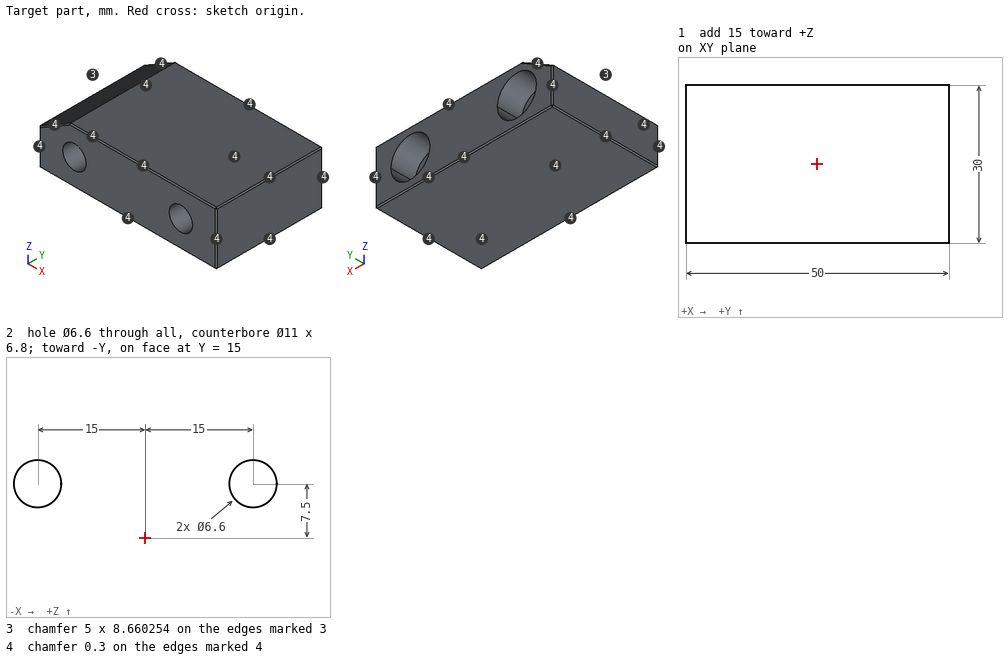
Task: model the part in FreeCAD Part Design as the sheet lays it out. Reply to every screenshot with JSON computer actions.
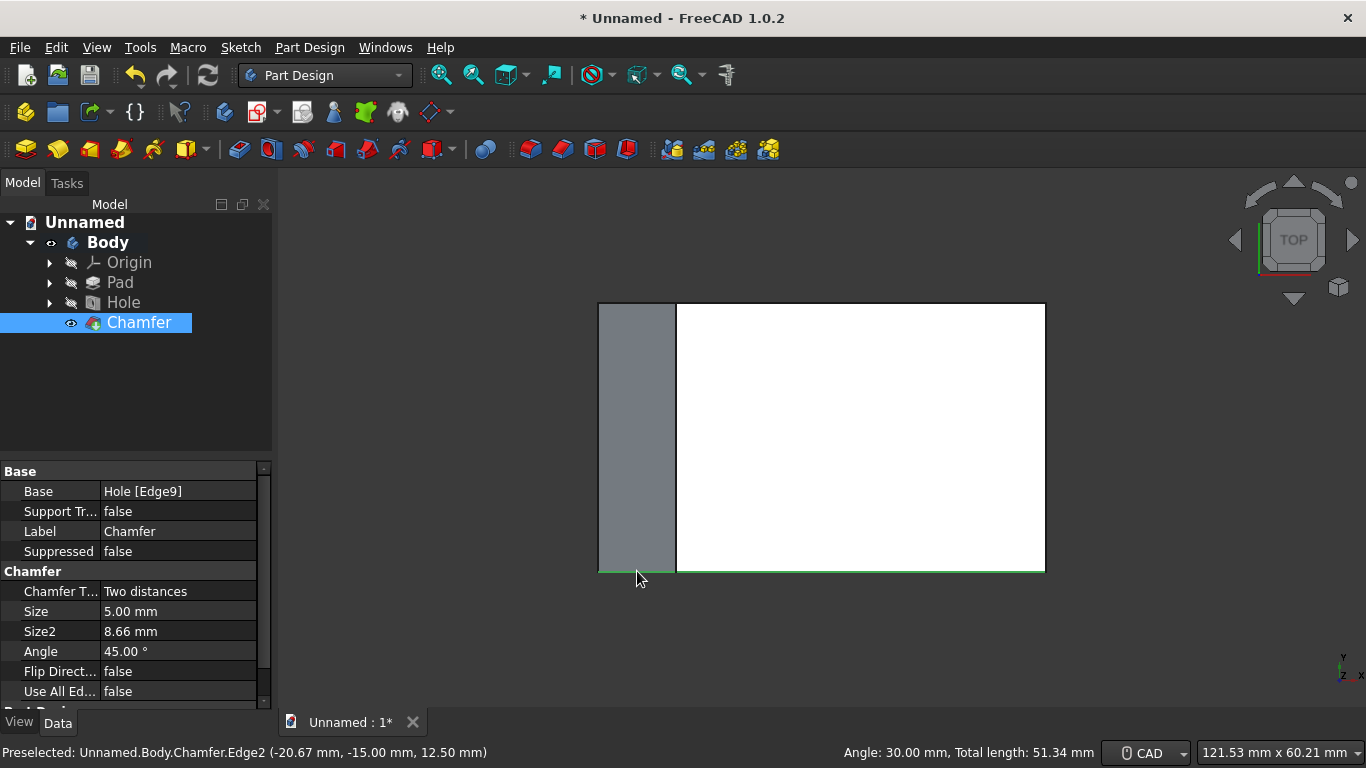
{"action": "left_click", "coordinate": [637, 302], "text": "ctrl"}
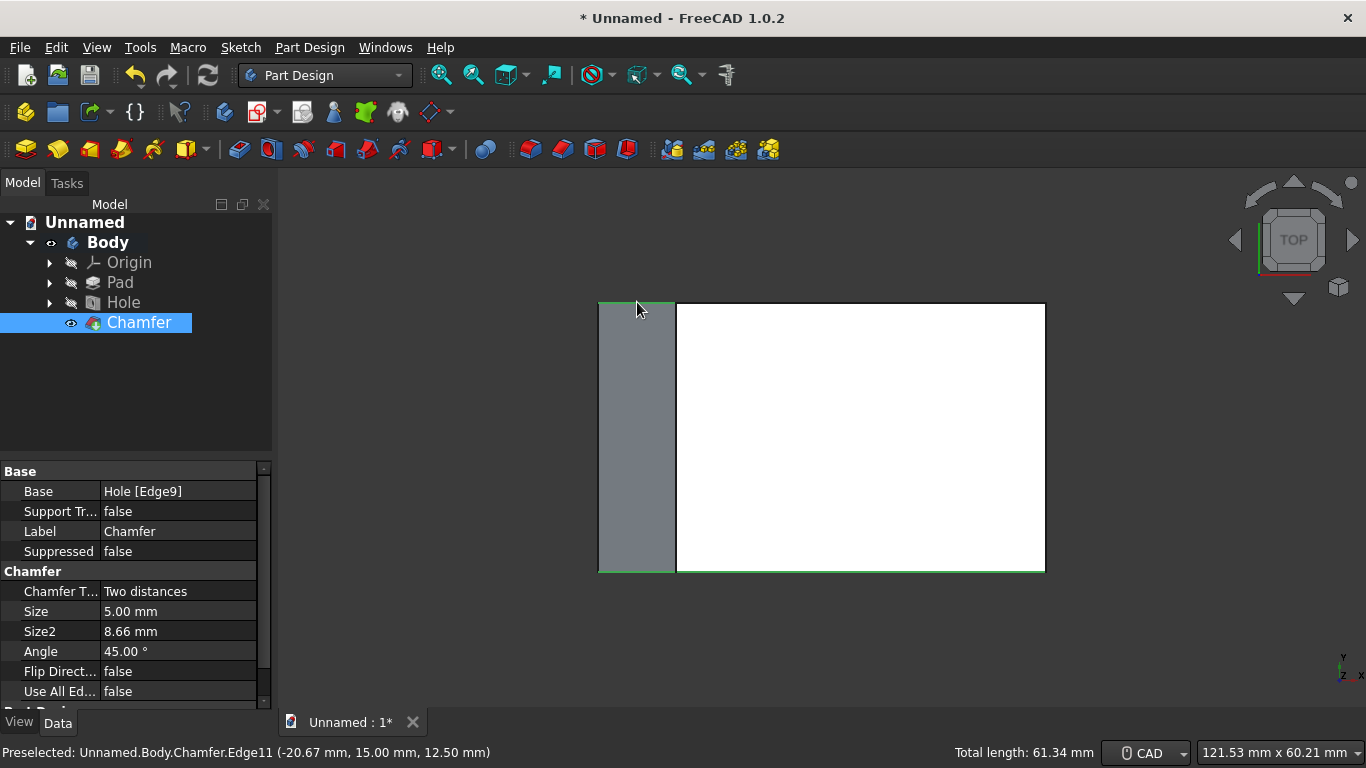
{"action": "left_click", "coordinate": [861, 302], "text": "ctrl"}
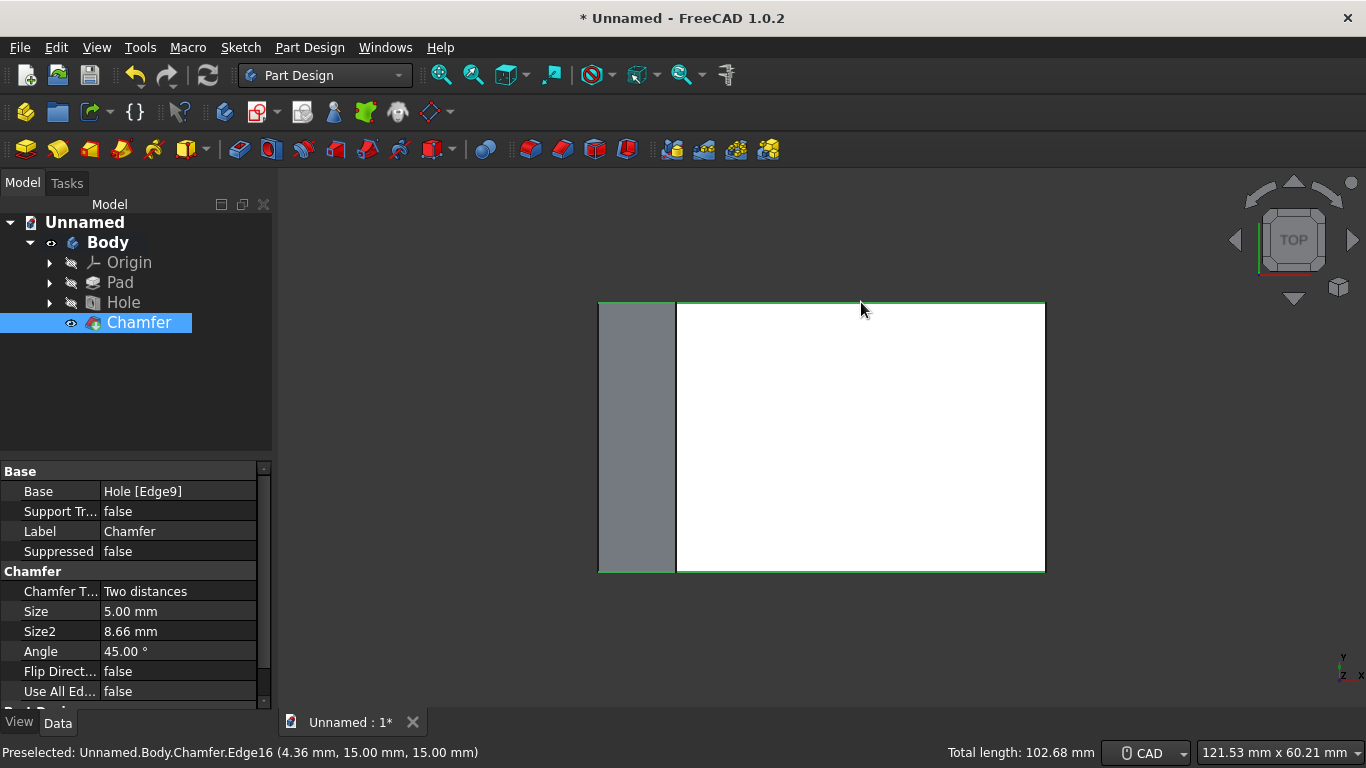
{"action": "key", "text": "0"}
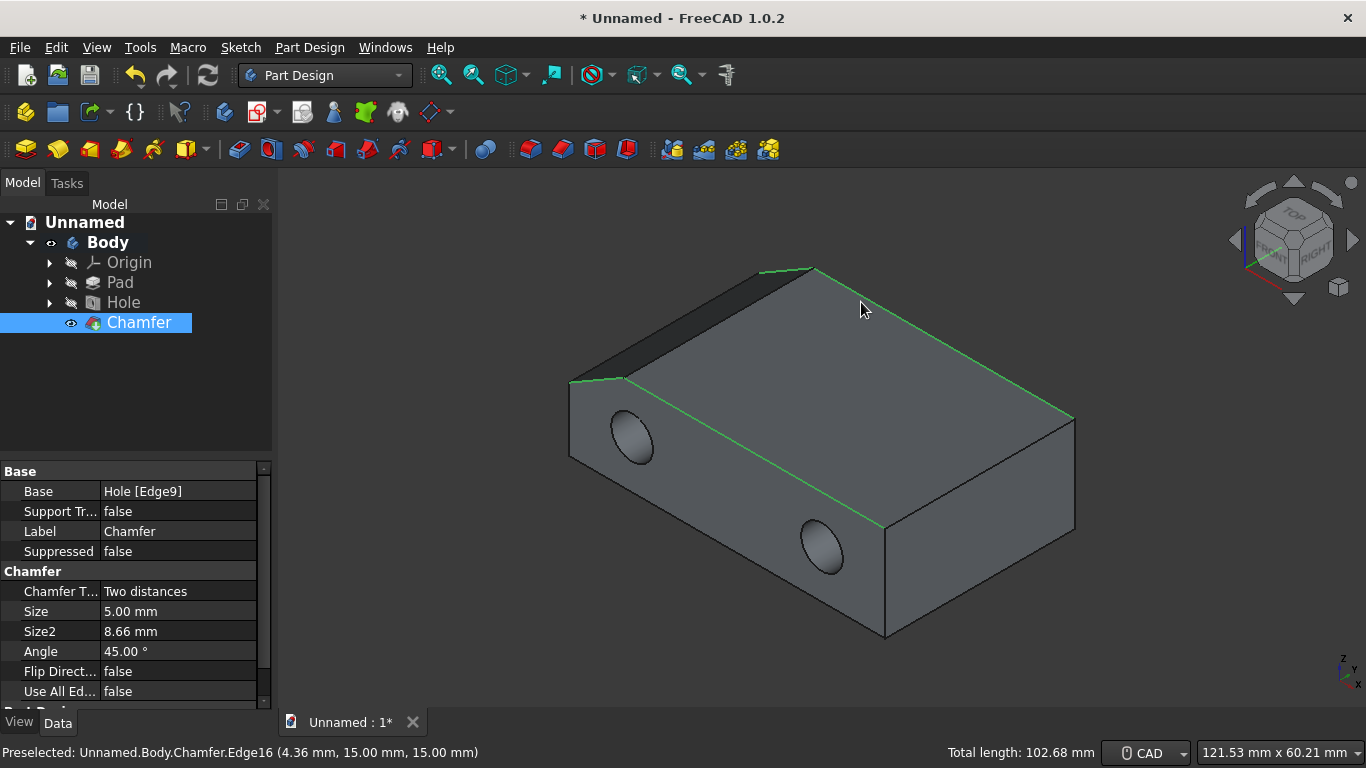
{"action": "left_click", "coordinate": [1007, 512], "text": "ctrl"}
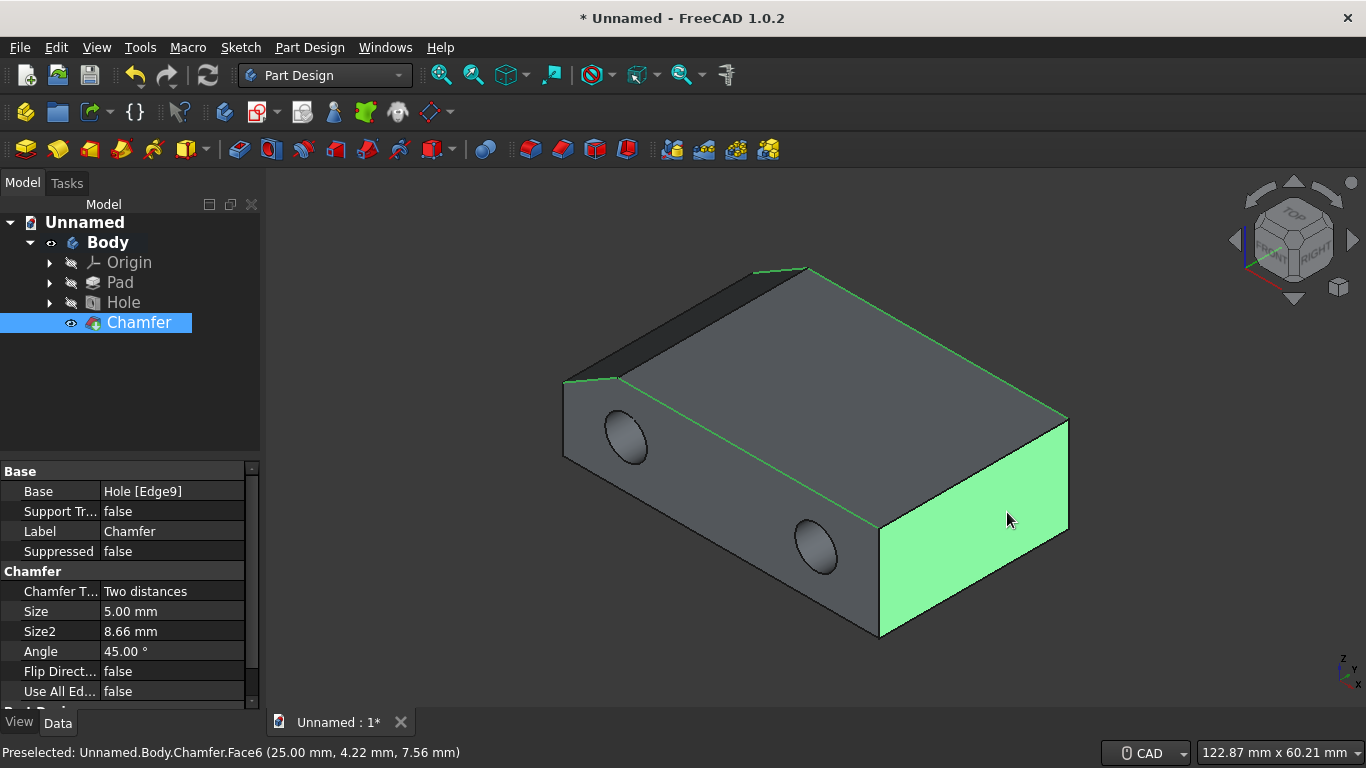
{"action": "key", "text": "2"}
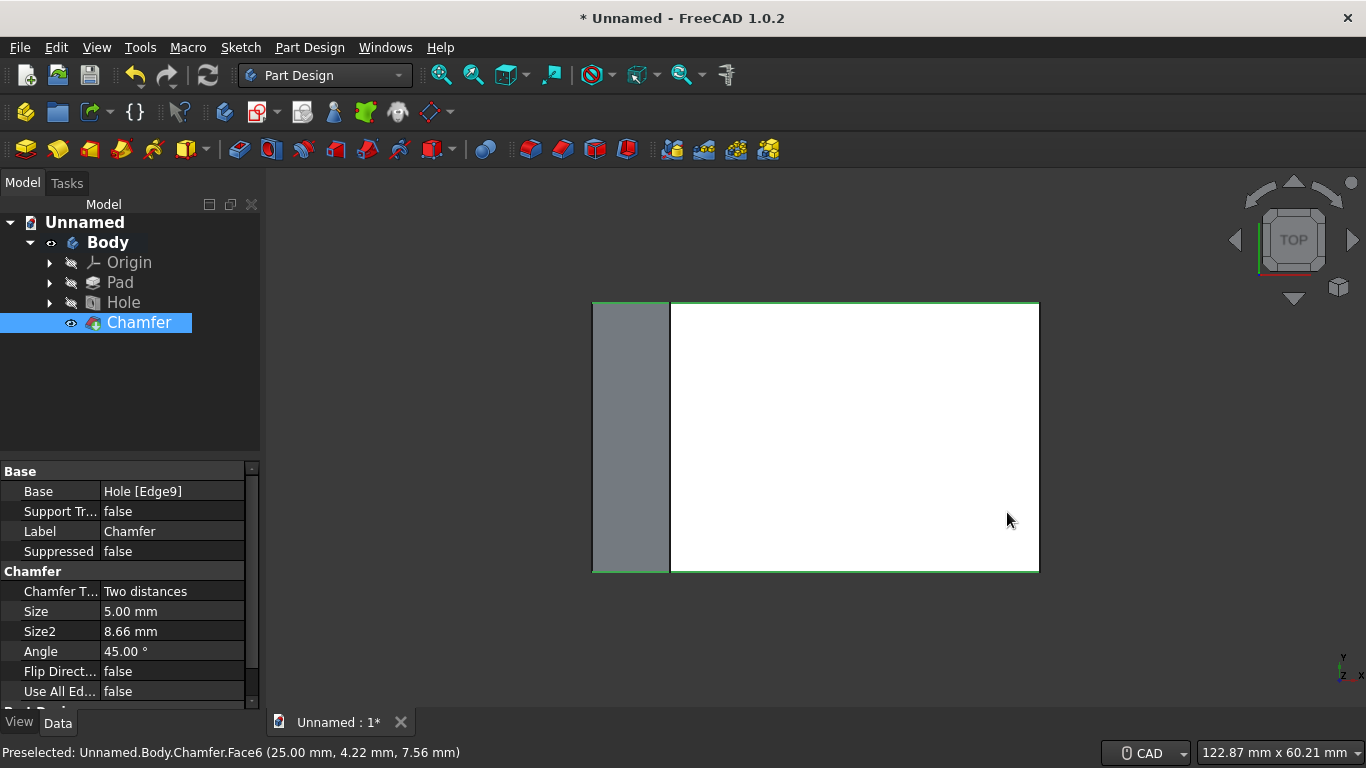
{"action": "key", "text": "1"}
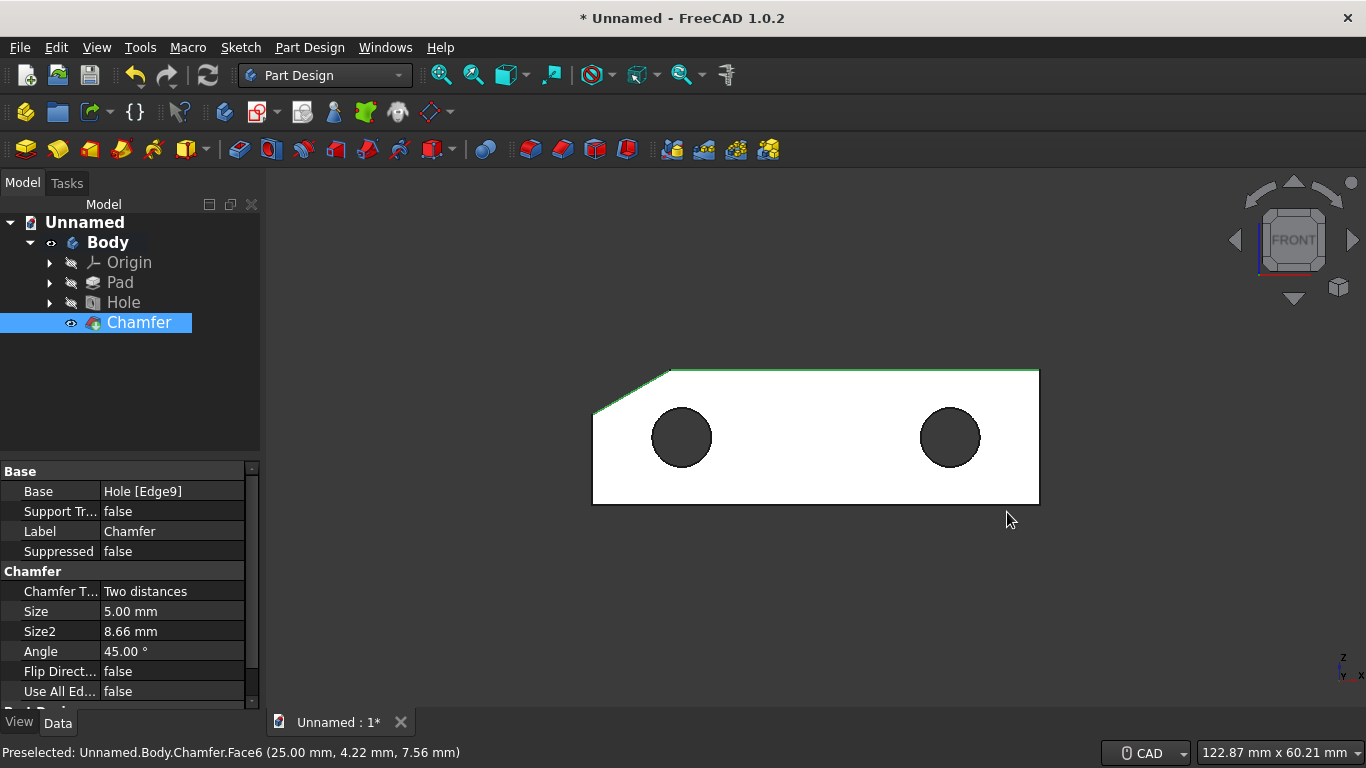
{"action": "left_click", "coordinate": [442, 76]}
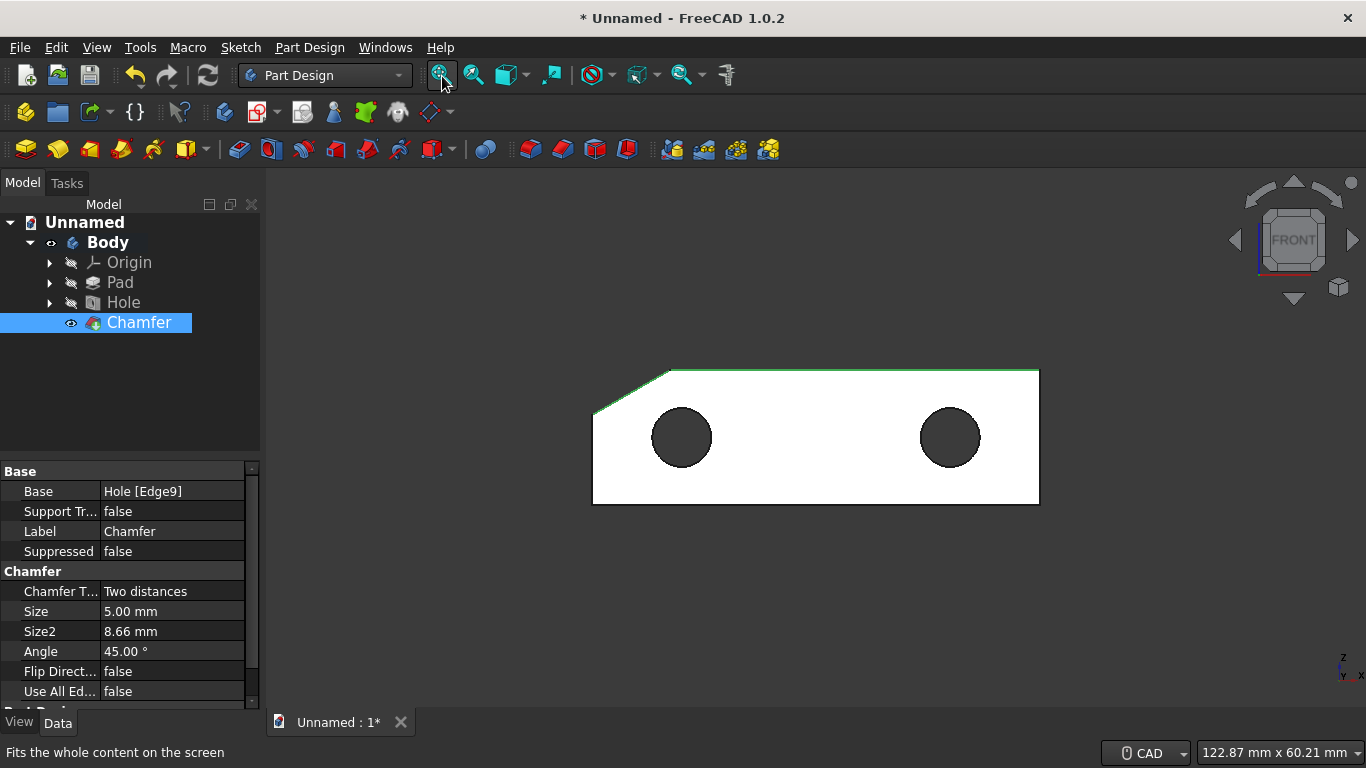
{"action": "left_click", "coordinate": [592, 459], "text": "ctrl"}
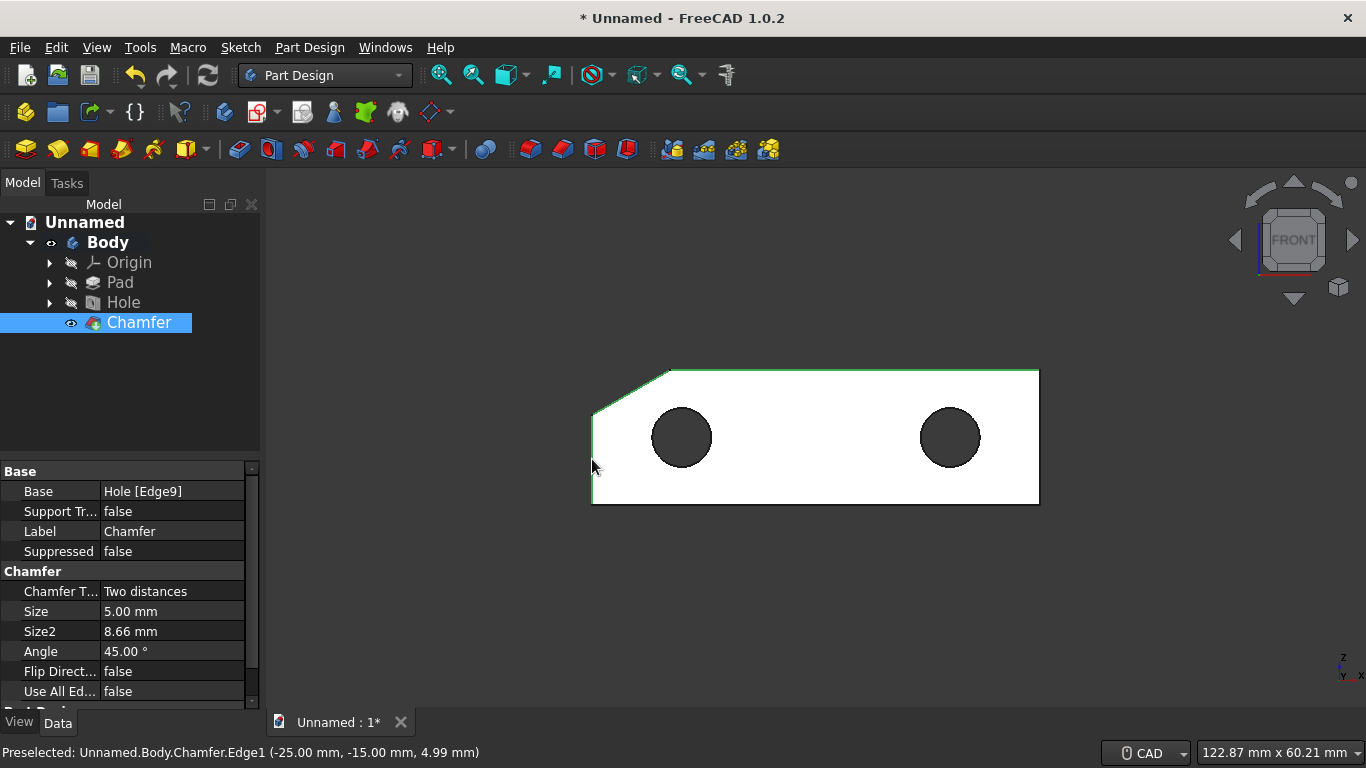
{"action": "key", "text": "3"}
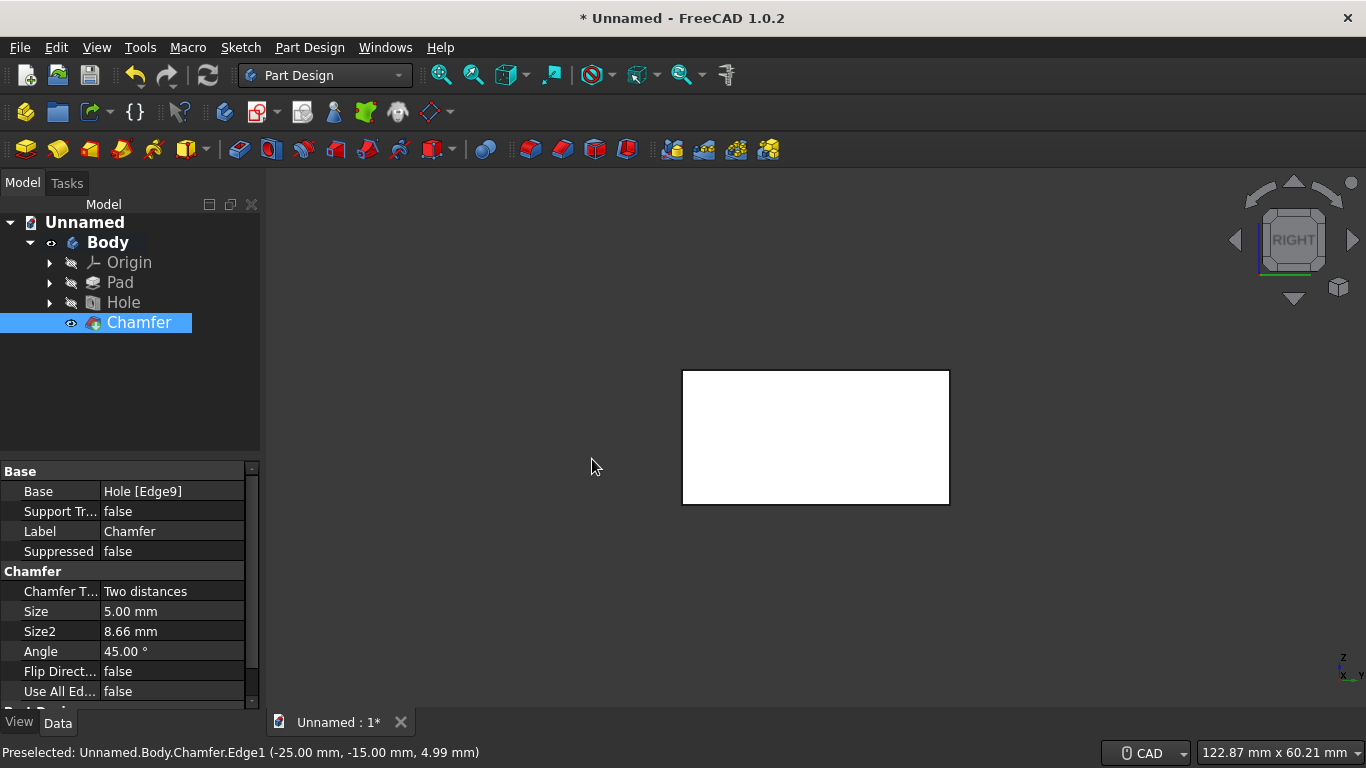
{"action": "left_click", "coordinate": [442, 76]}